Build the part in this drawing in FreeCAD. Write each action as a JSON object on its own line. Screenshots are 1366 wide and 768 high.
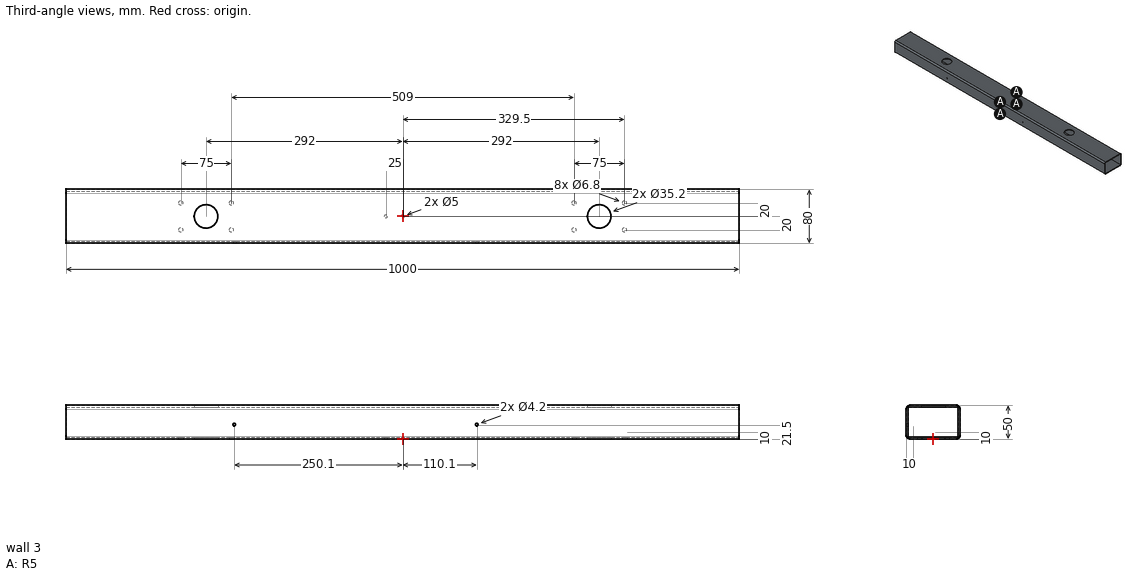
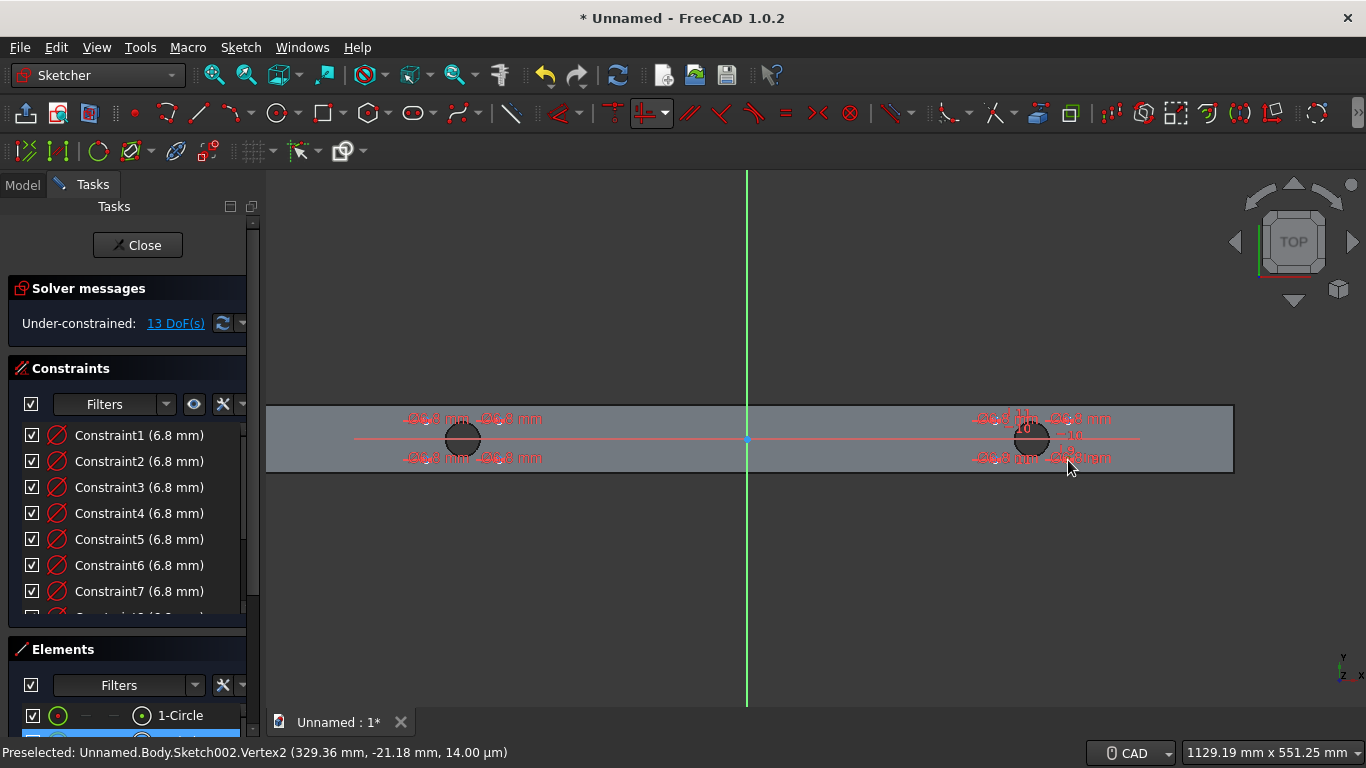
{"action": "left_click", "coordinate": [995, 460]}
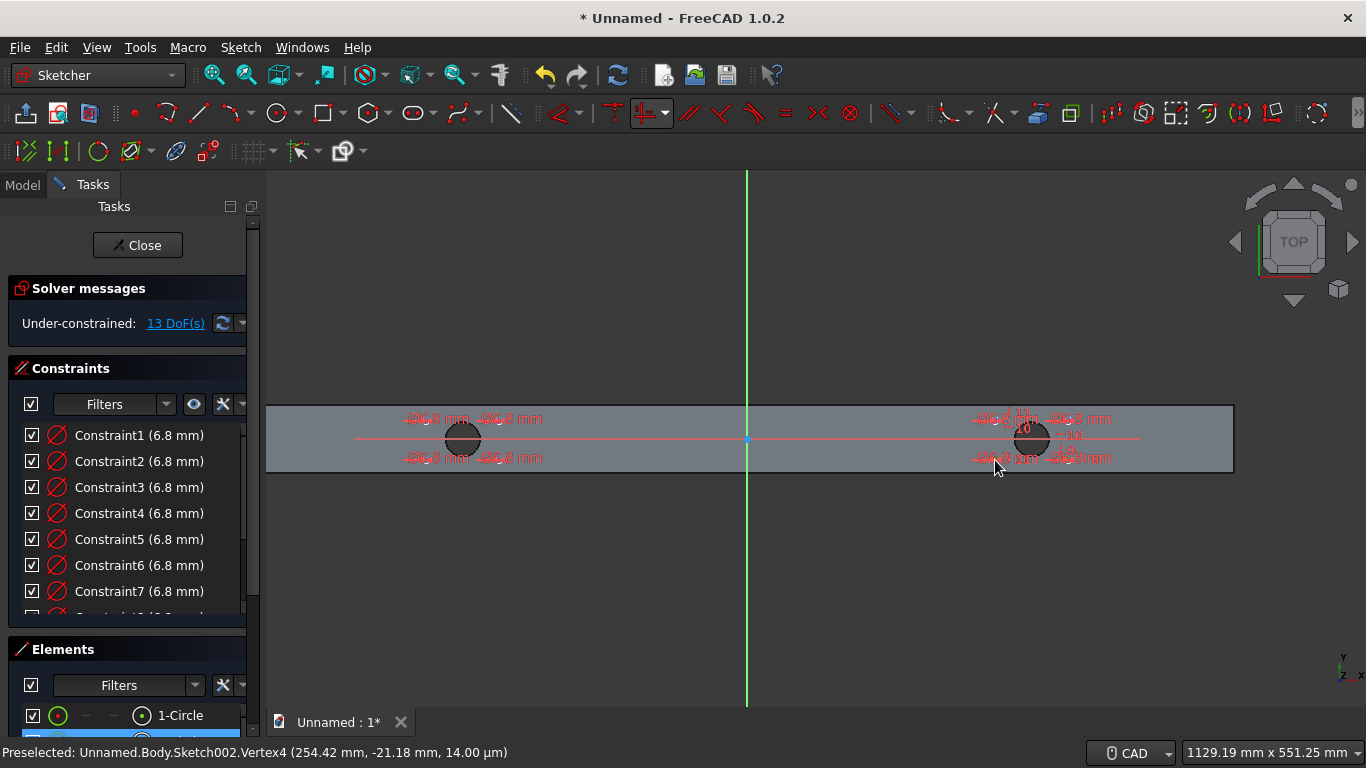
{"action": "left_click", "coordinate": [668, 114]}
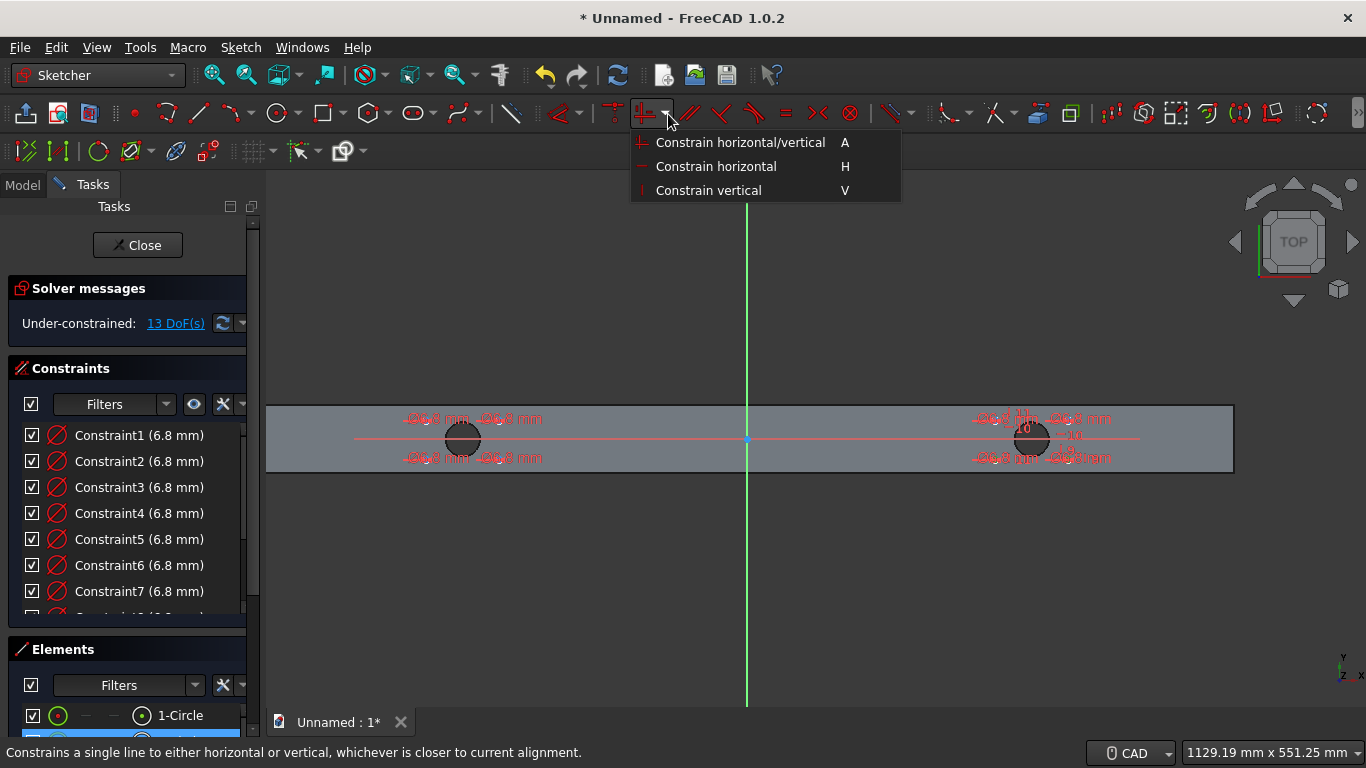
{"action": "left_click", "coordinate": [766, 166]}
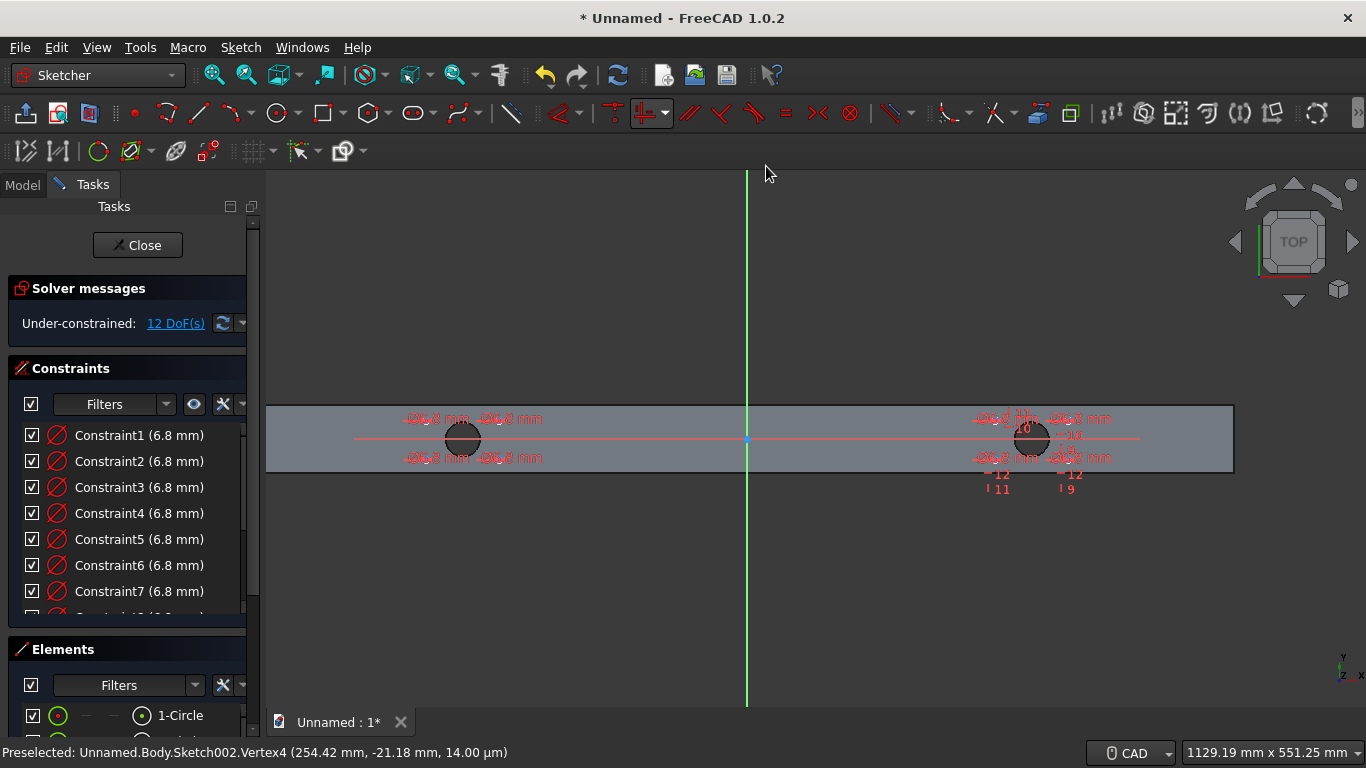
{"action": "left_click", "coordinate": [995, 421]}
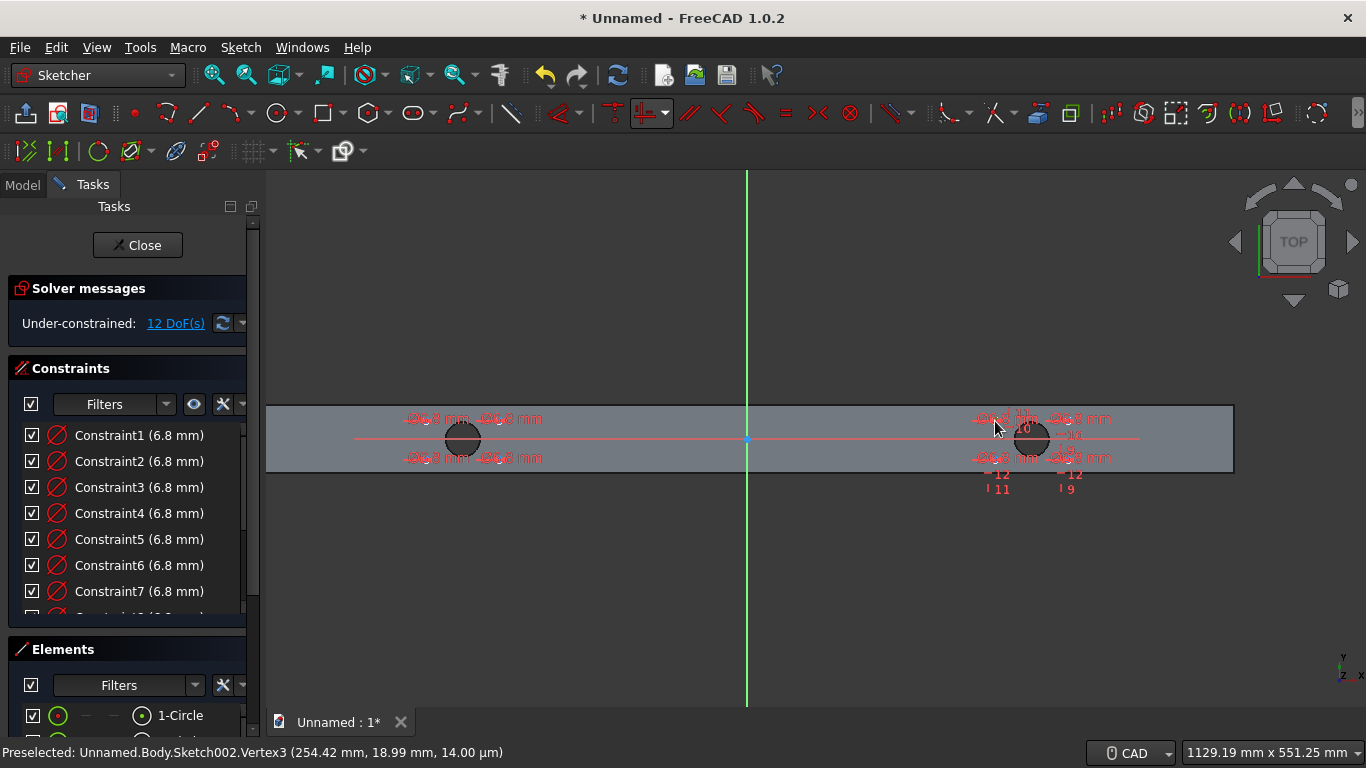
{"action": "left_click", "coordinate": [499, 421]}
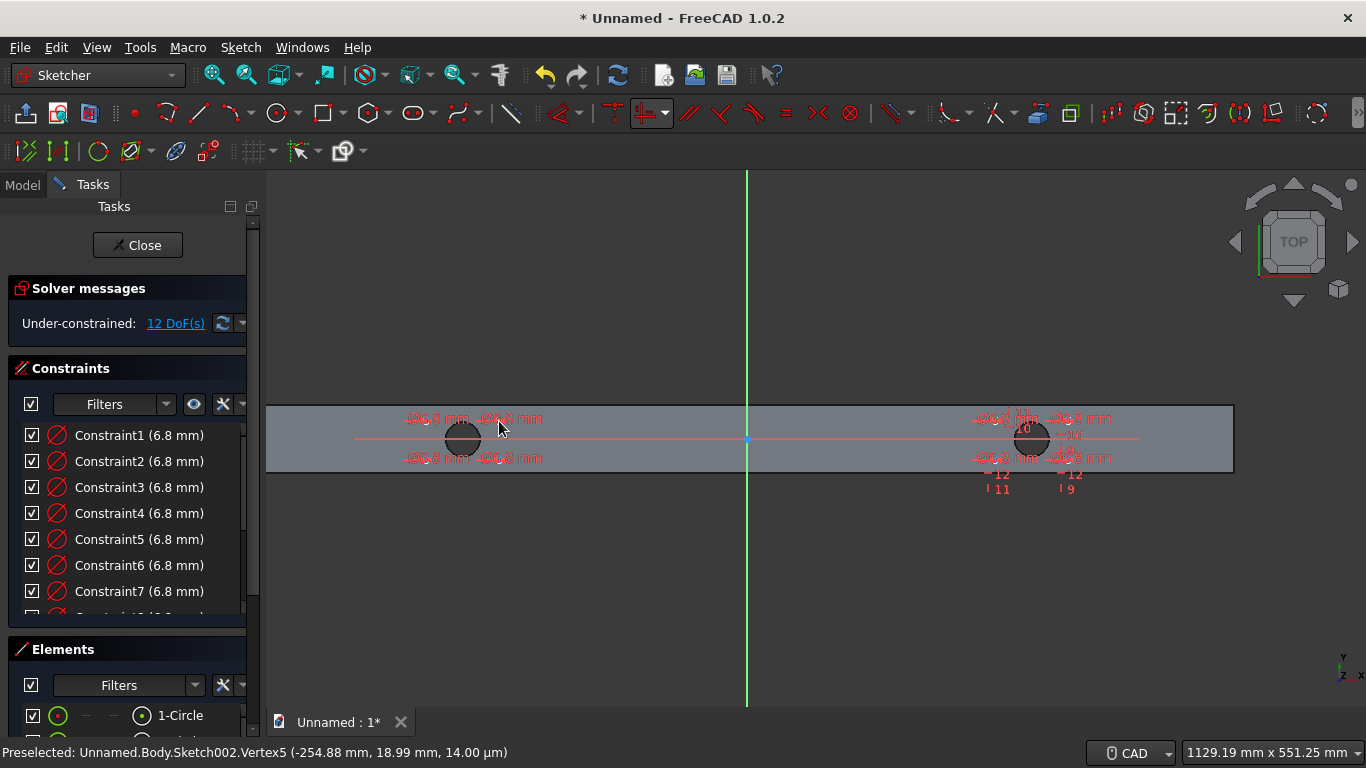
{"action": "left_click", "coordinate": [668, 114]}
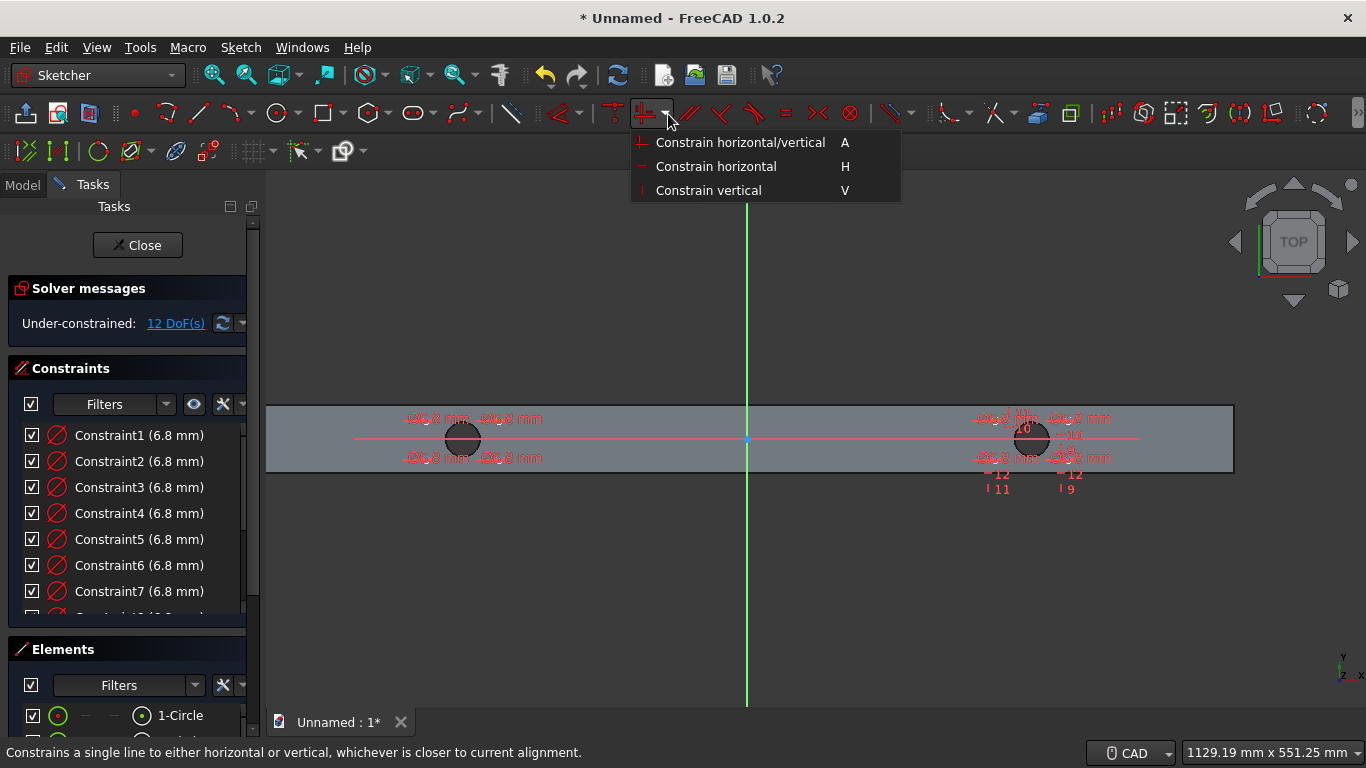
{"action": "left_click", "coordinate": [766, 166]}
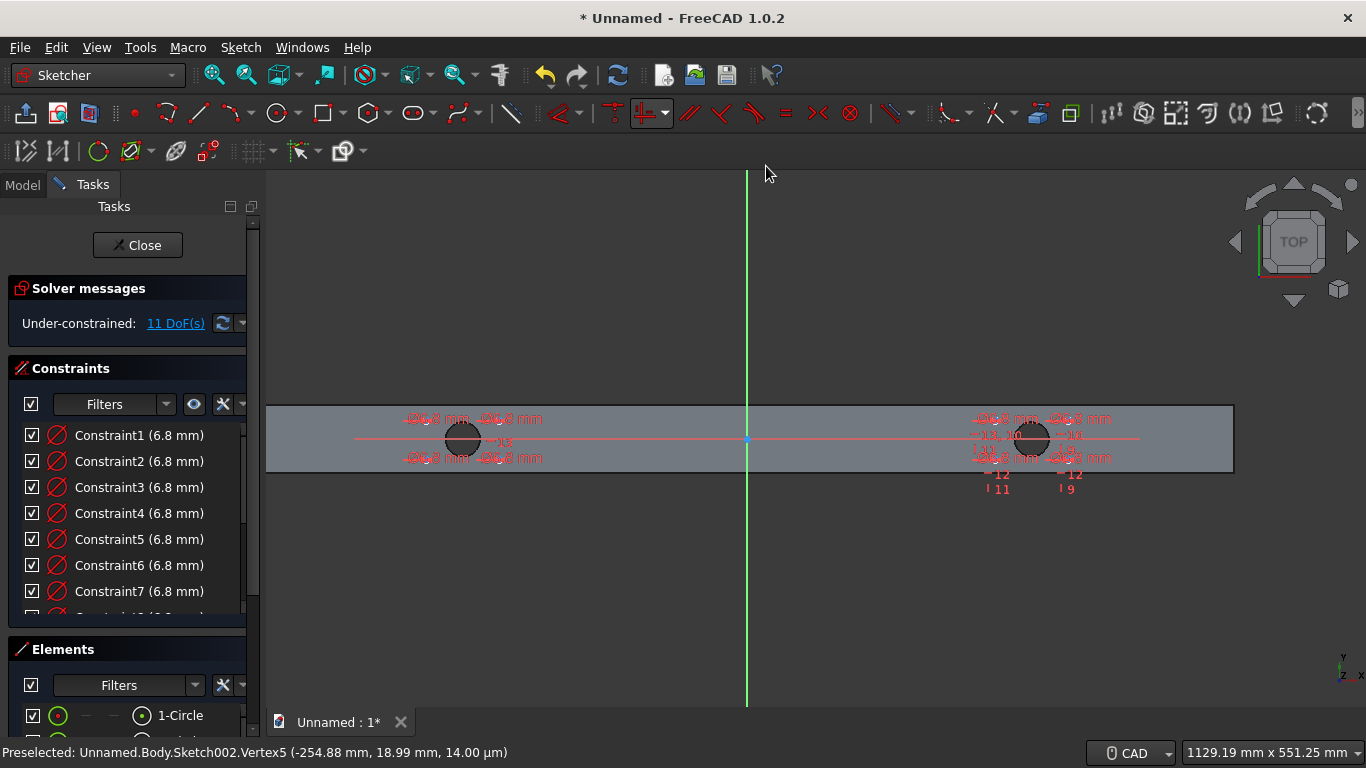
{"action": "left_click", "coordinate": [499, 421]}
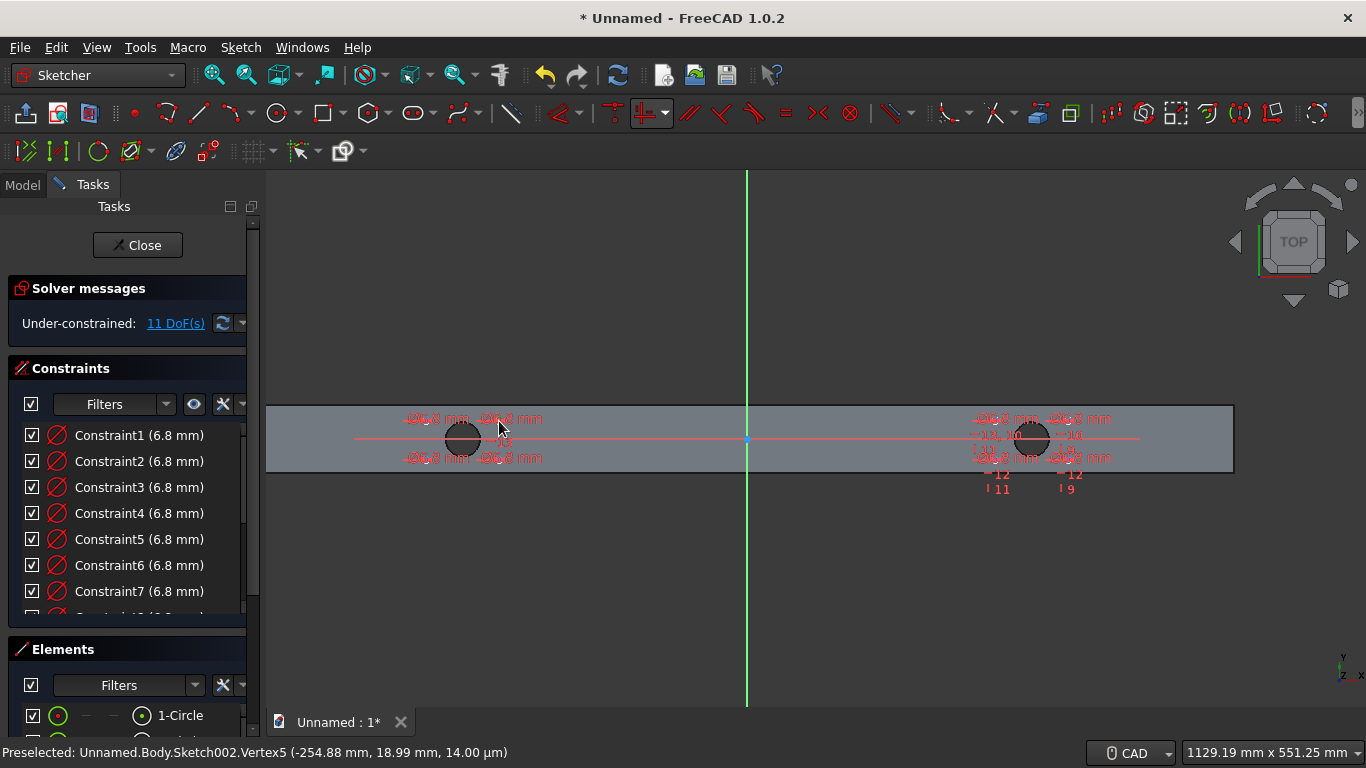
{"action": "left_click", "coordinate": [499, 460]}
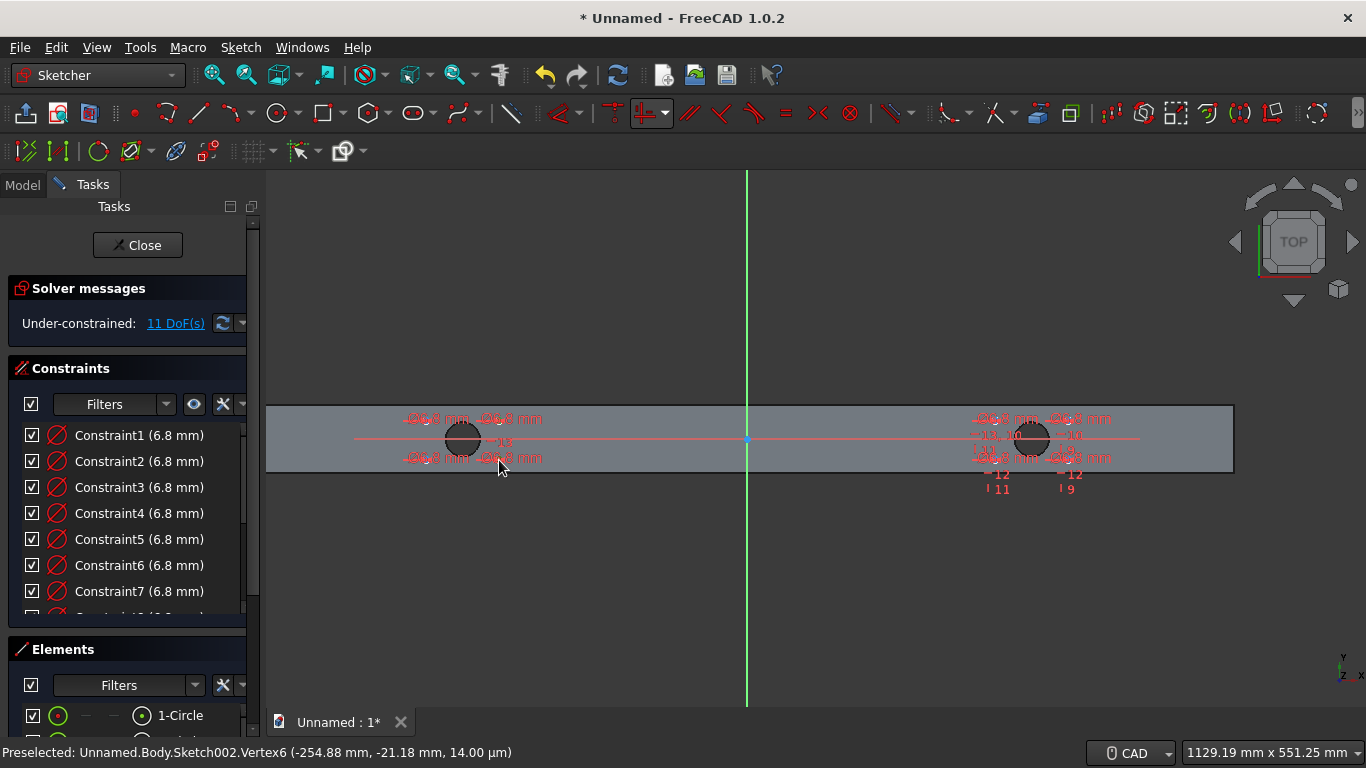
{"action": "key", "text": "v"}